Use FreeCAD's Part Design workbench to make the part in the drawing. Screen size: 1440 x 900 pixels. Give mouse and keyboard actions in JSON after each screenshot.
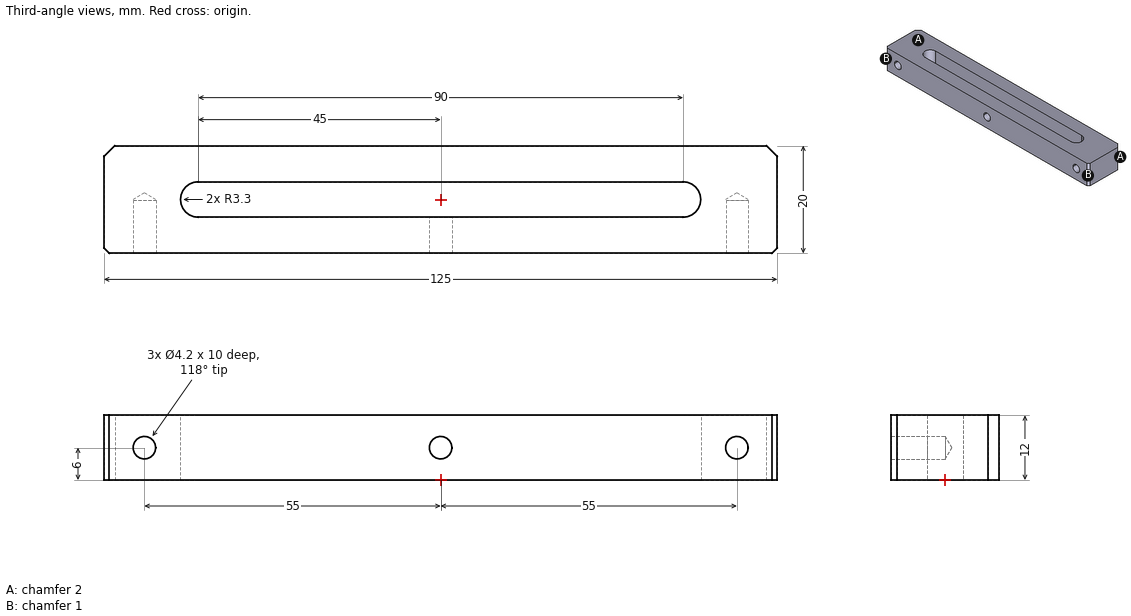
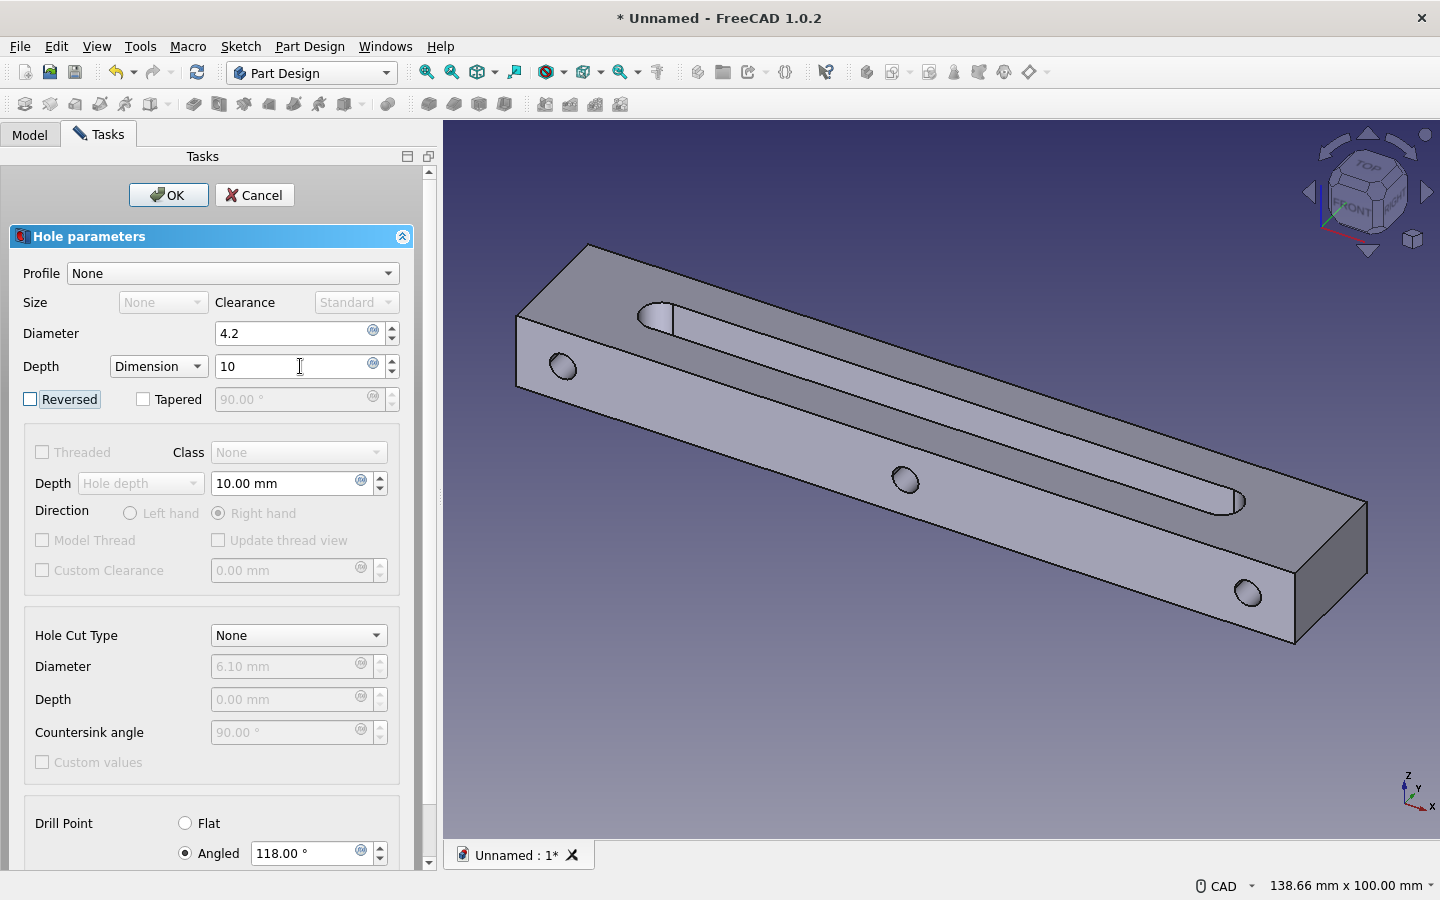
{"action": "left_click", "coordinate": [169, 195]}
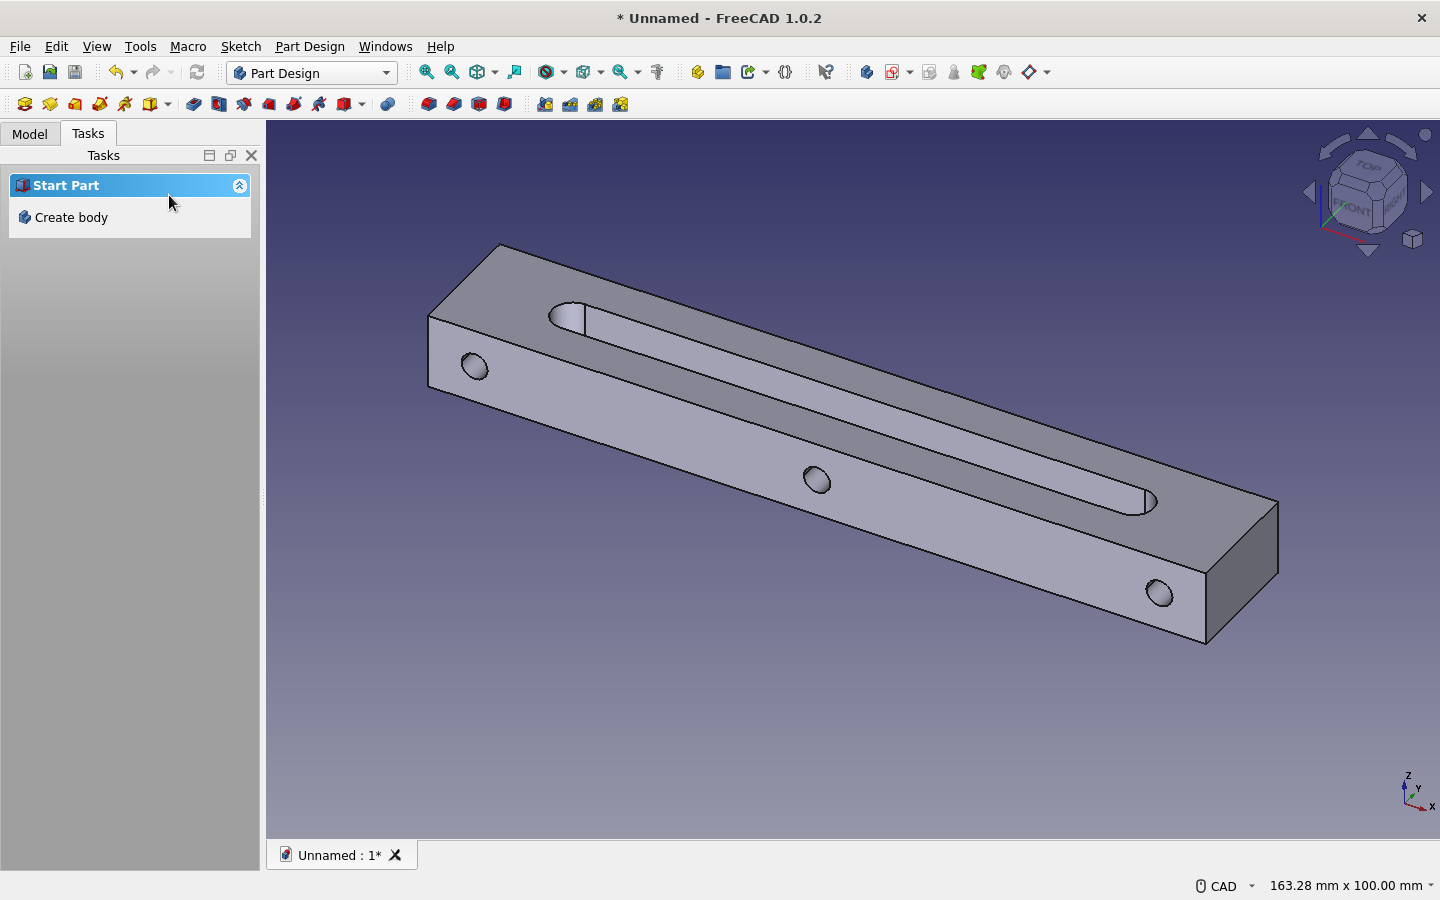
{"action": "key", "text": "0"}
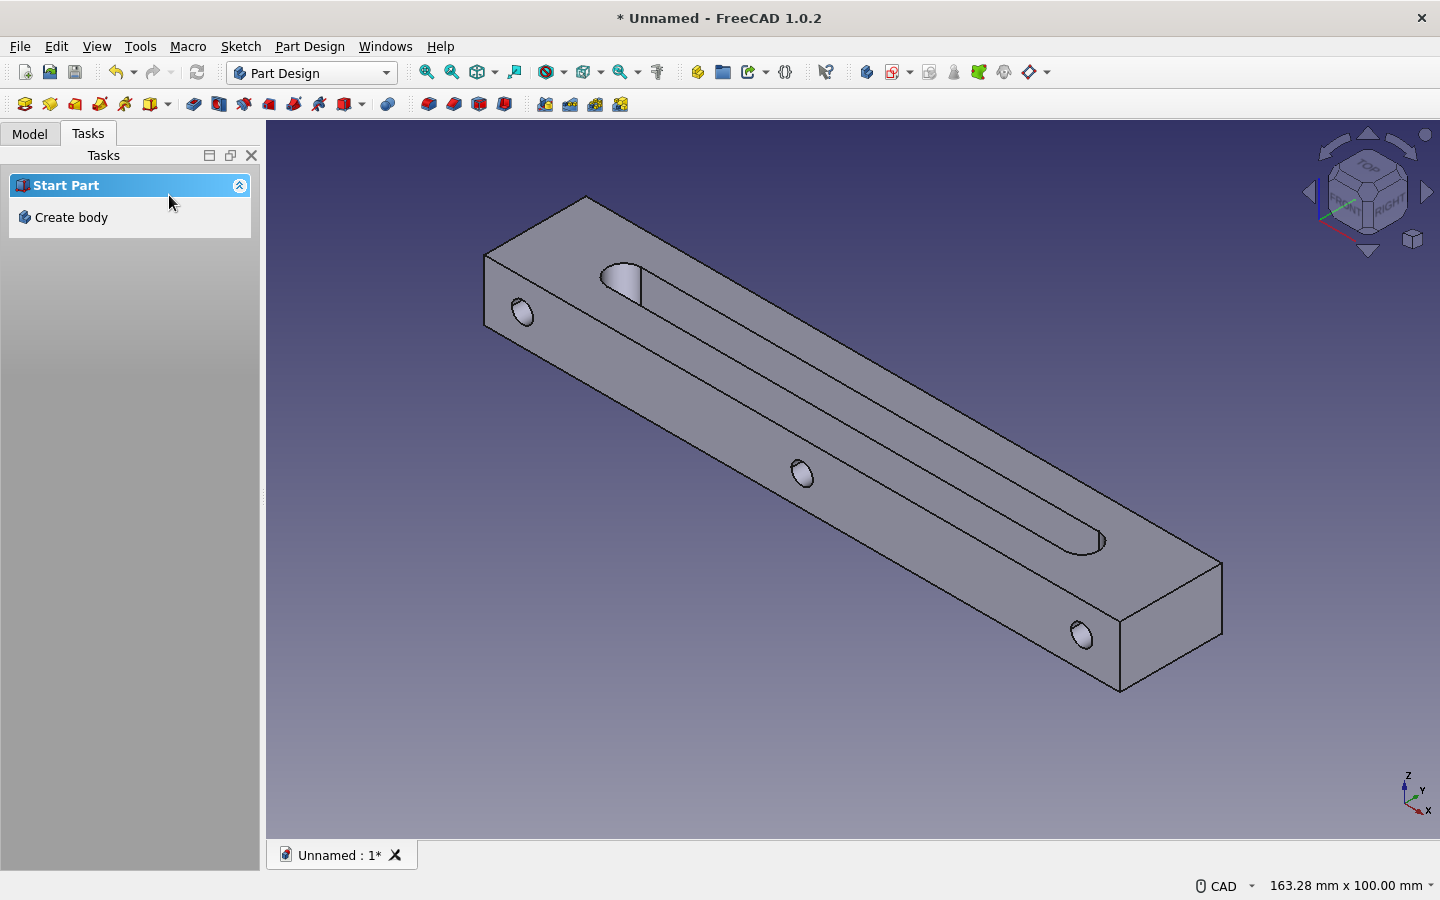
{"action": "key", "text": "2"}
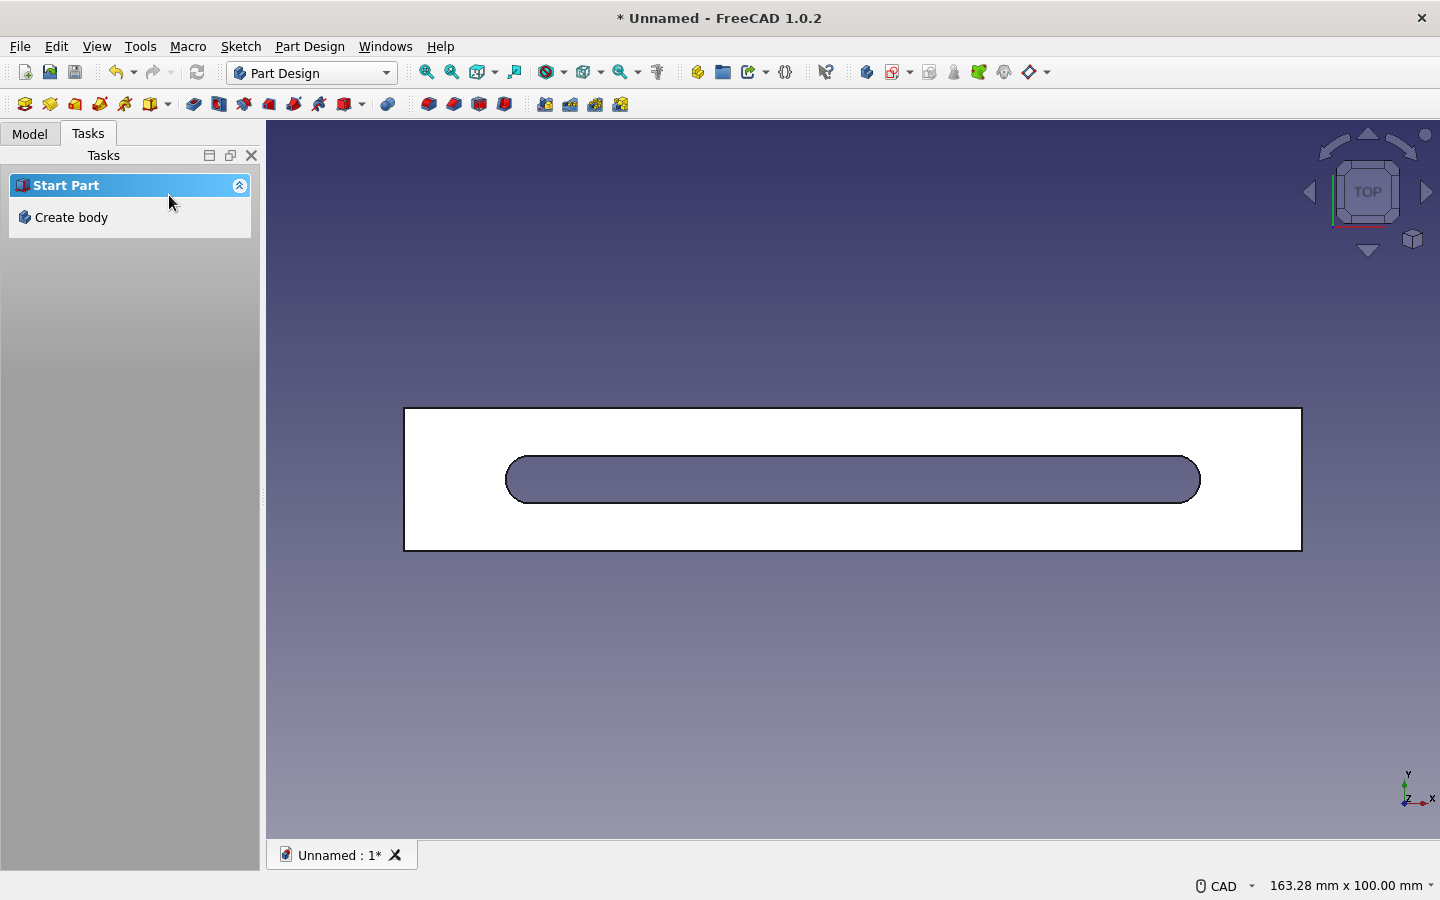
{"action": "key", "text": "1"}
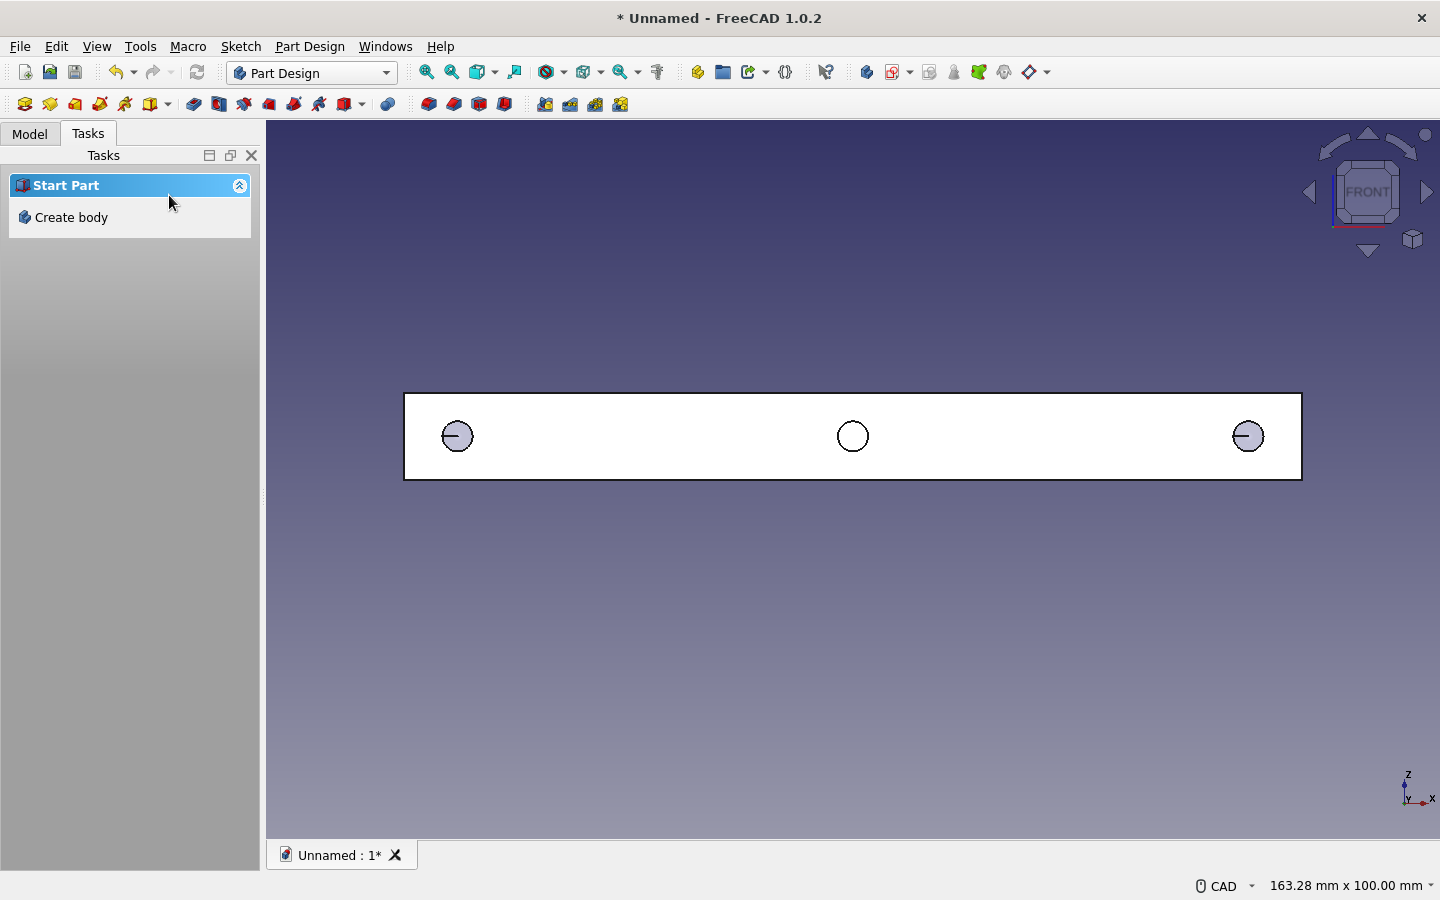
{"action": "key", "text": "3"}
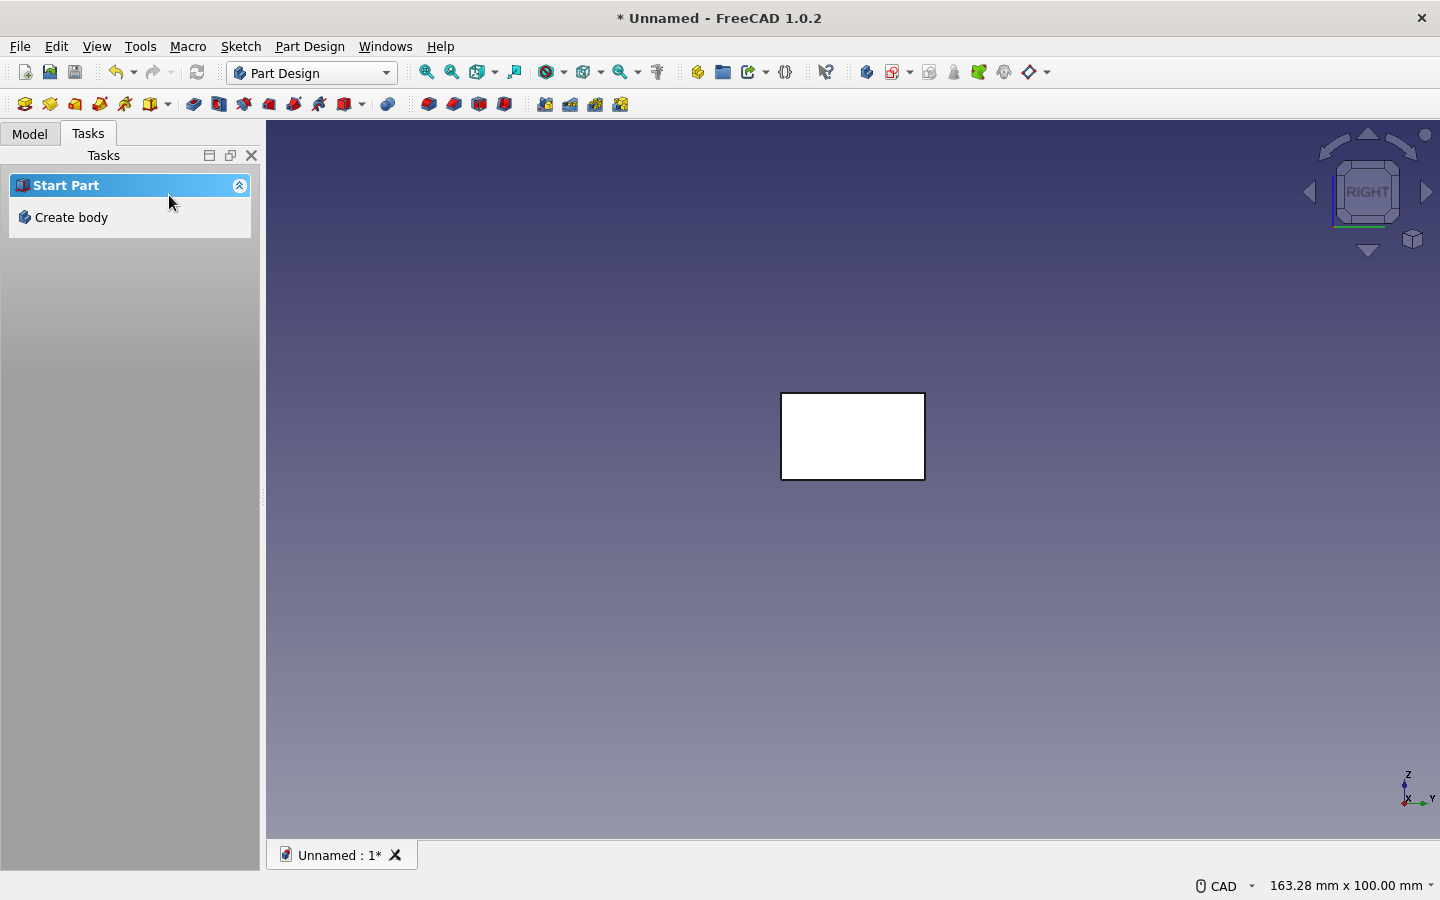
{"action": "left_click", "coordinate": [427, 72]}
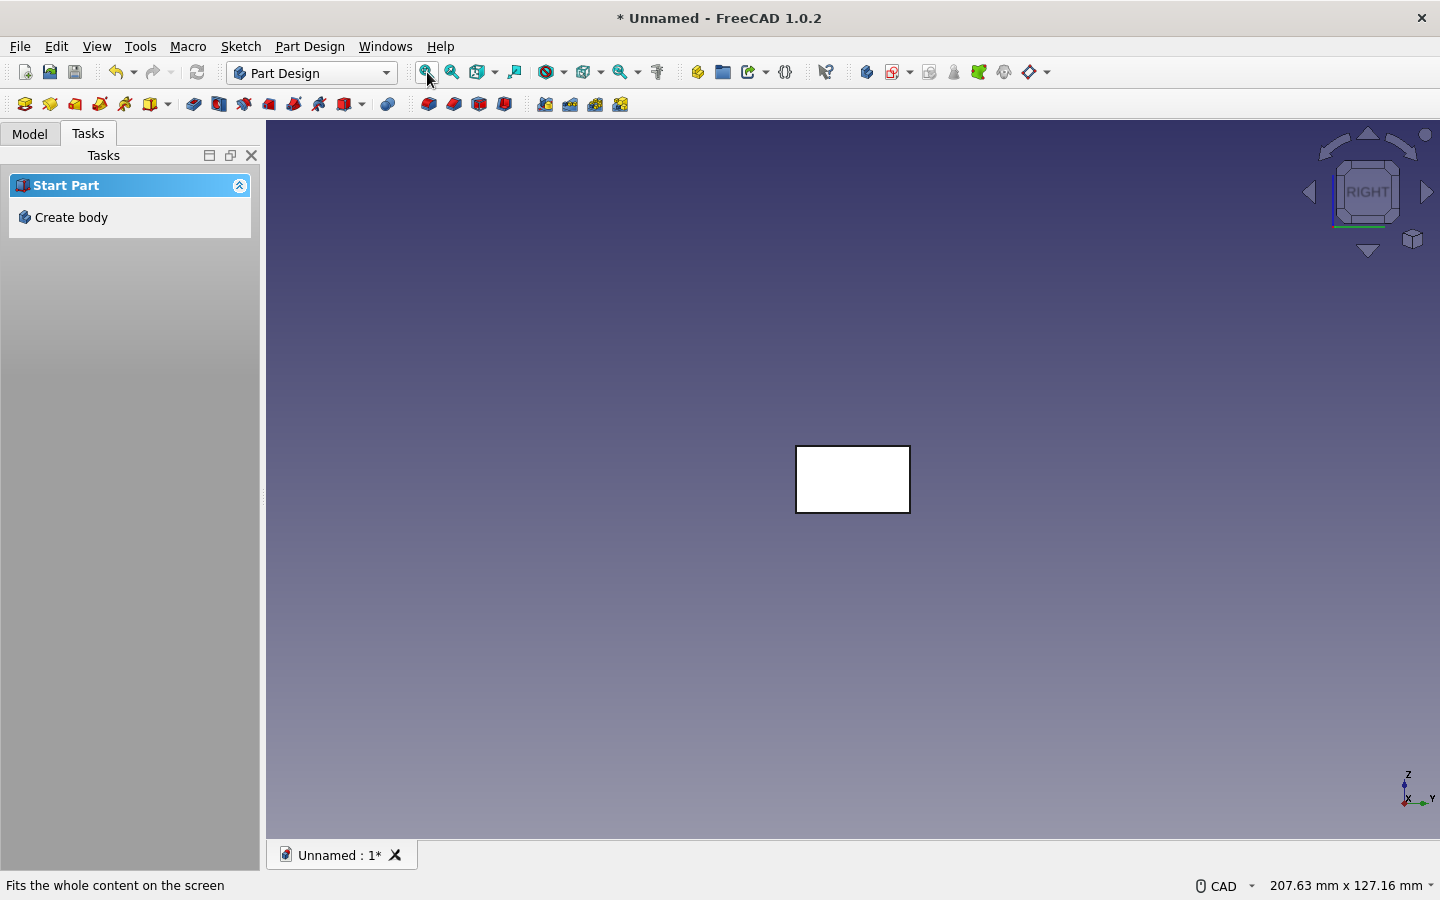
{"action": "left_click", "coordinate": [910, 478]}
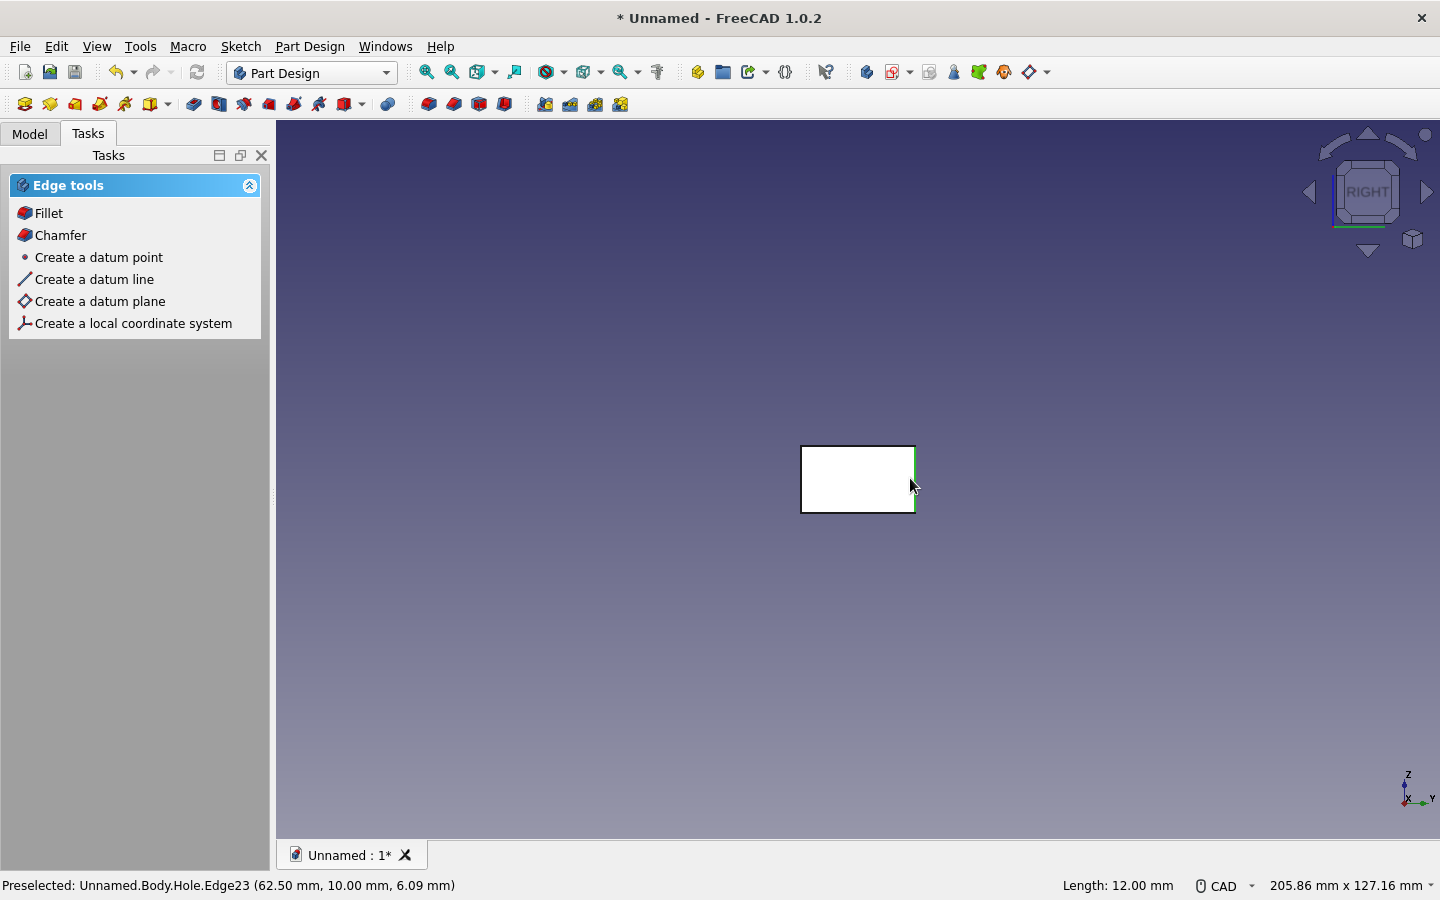
{"action": "key", "text": "5"}